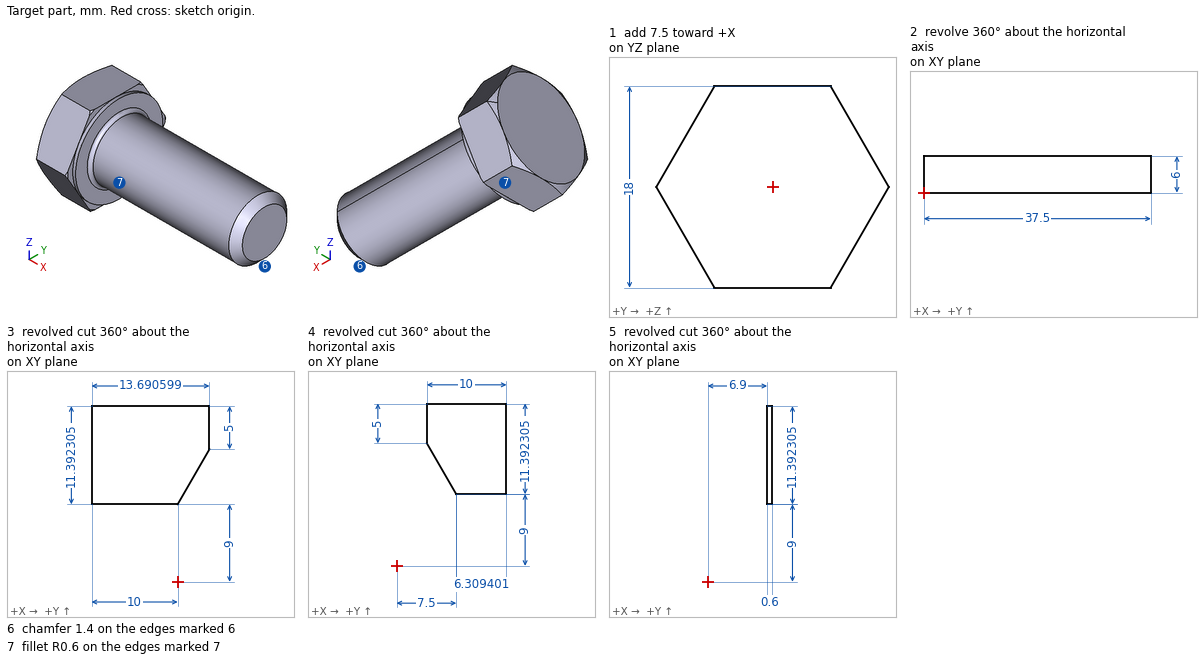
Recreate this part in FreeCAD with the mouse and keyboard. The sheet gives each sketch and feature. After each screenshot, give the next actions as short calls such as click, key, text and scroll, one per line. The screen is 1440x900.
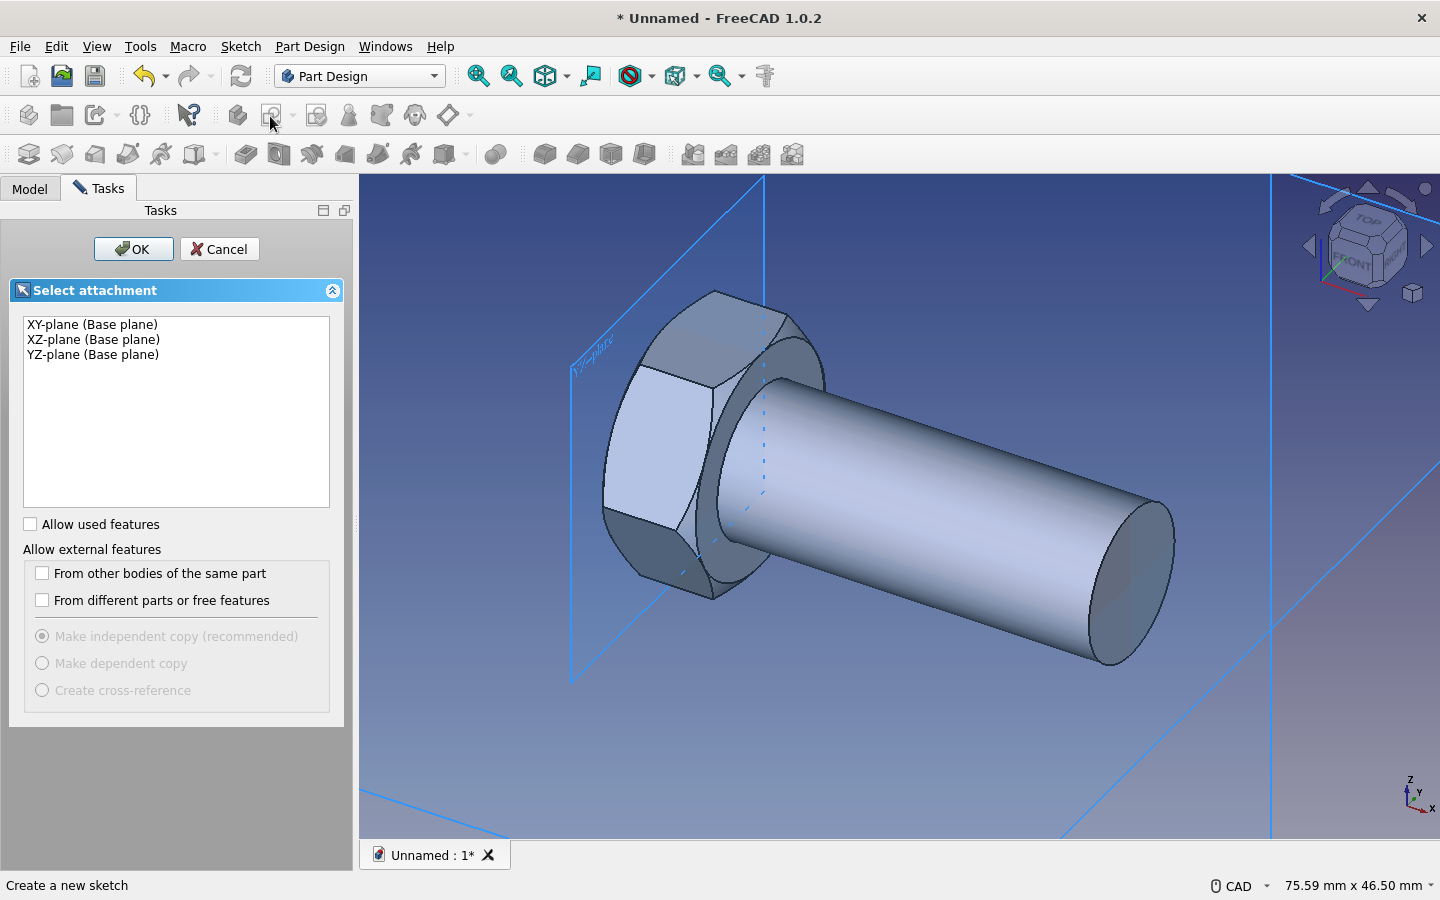
click(84, 324)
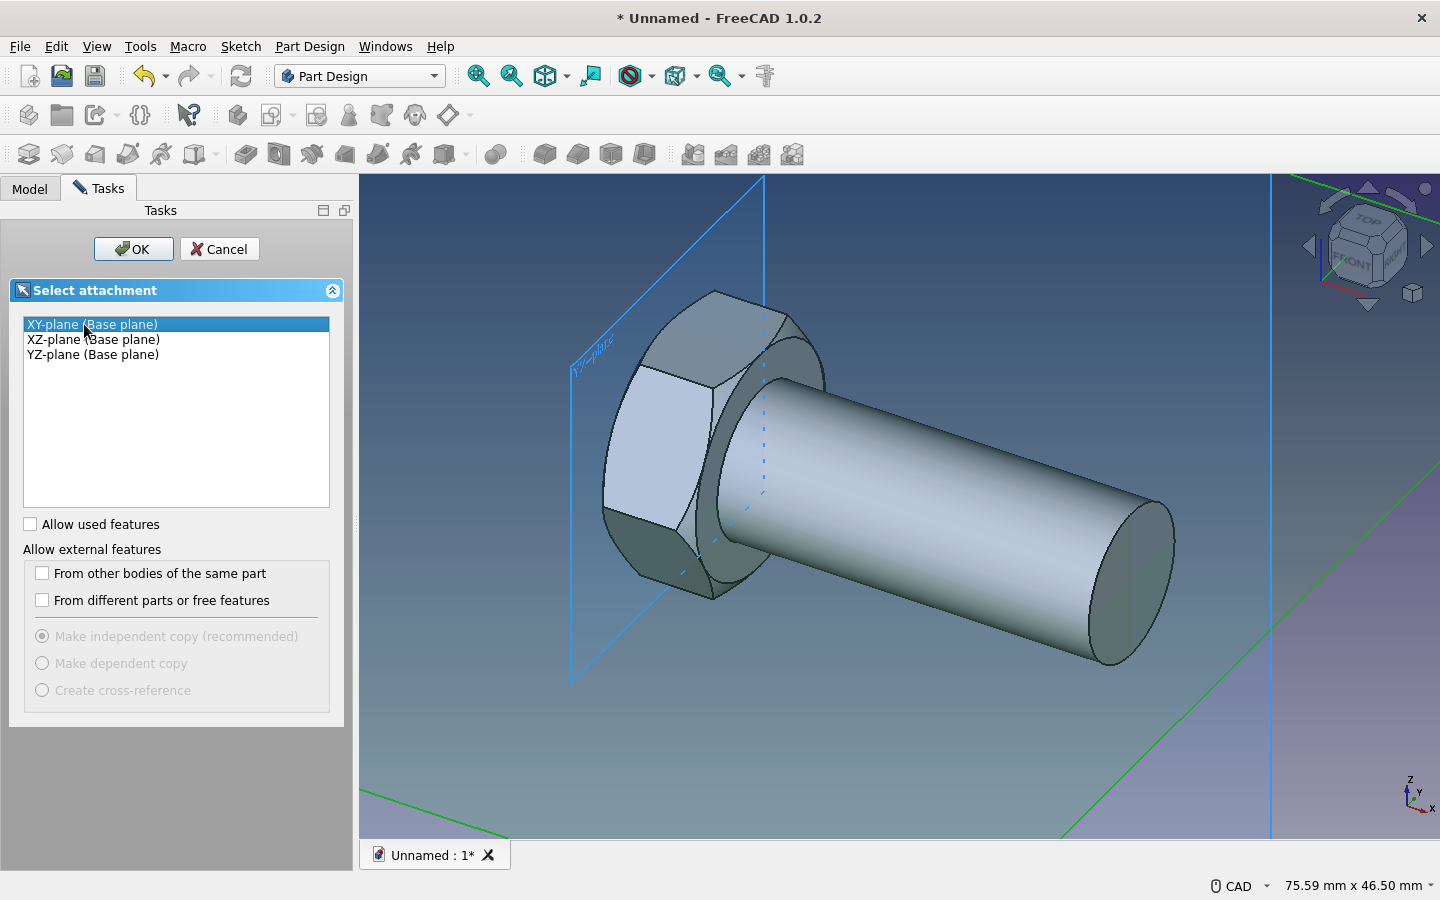
click(134, 249)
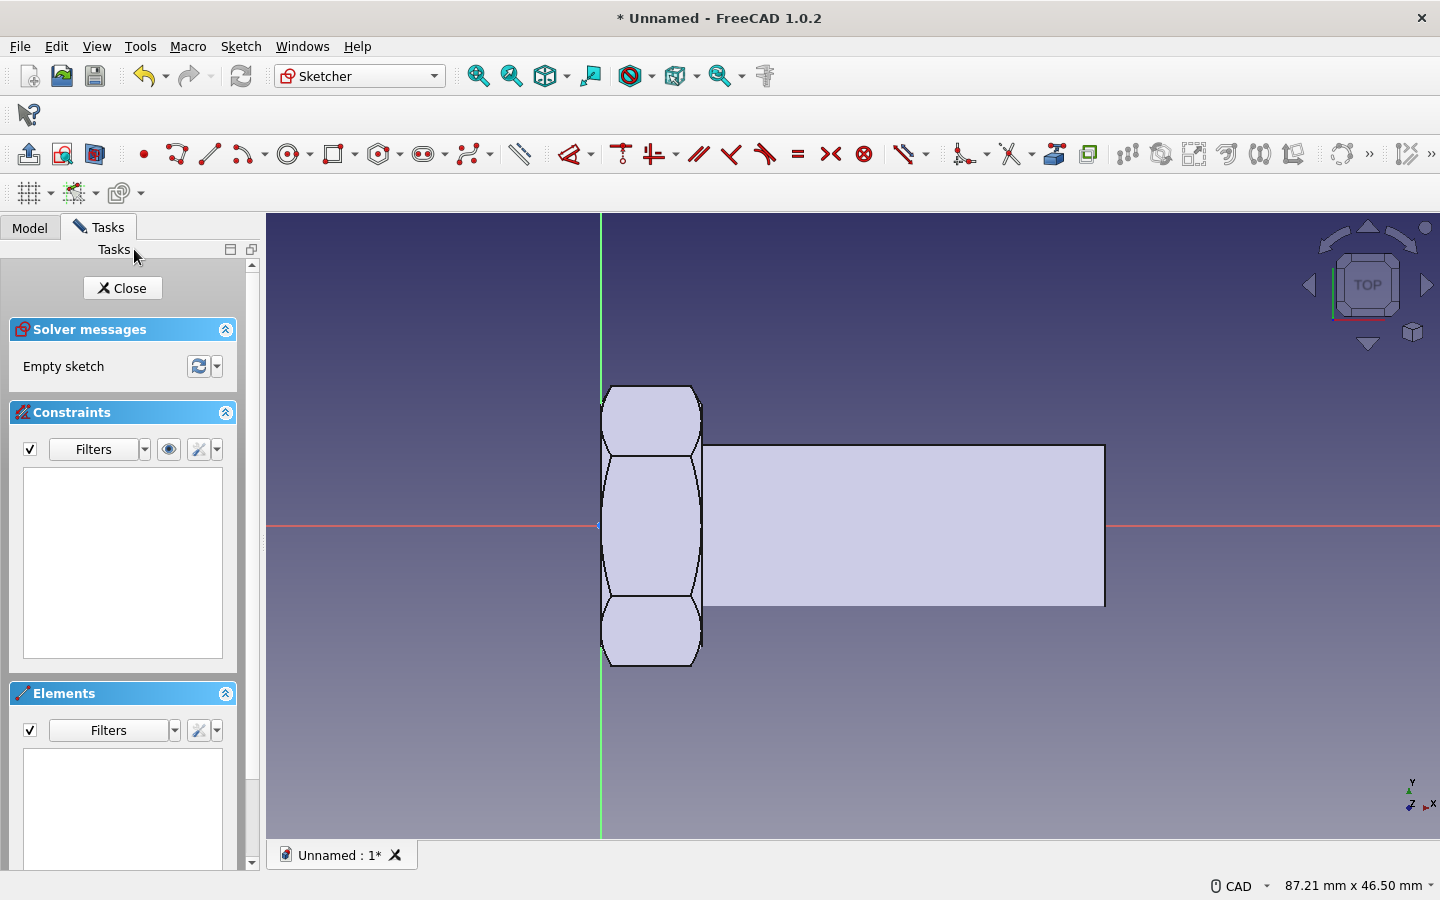
click(95, 154)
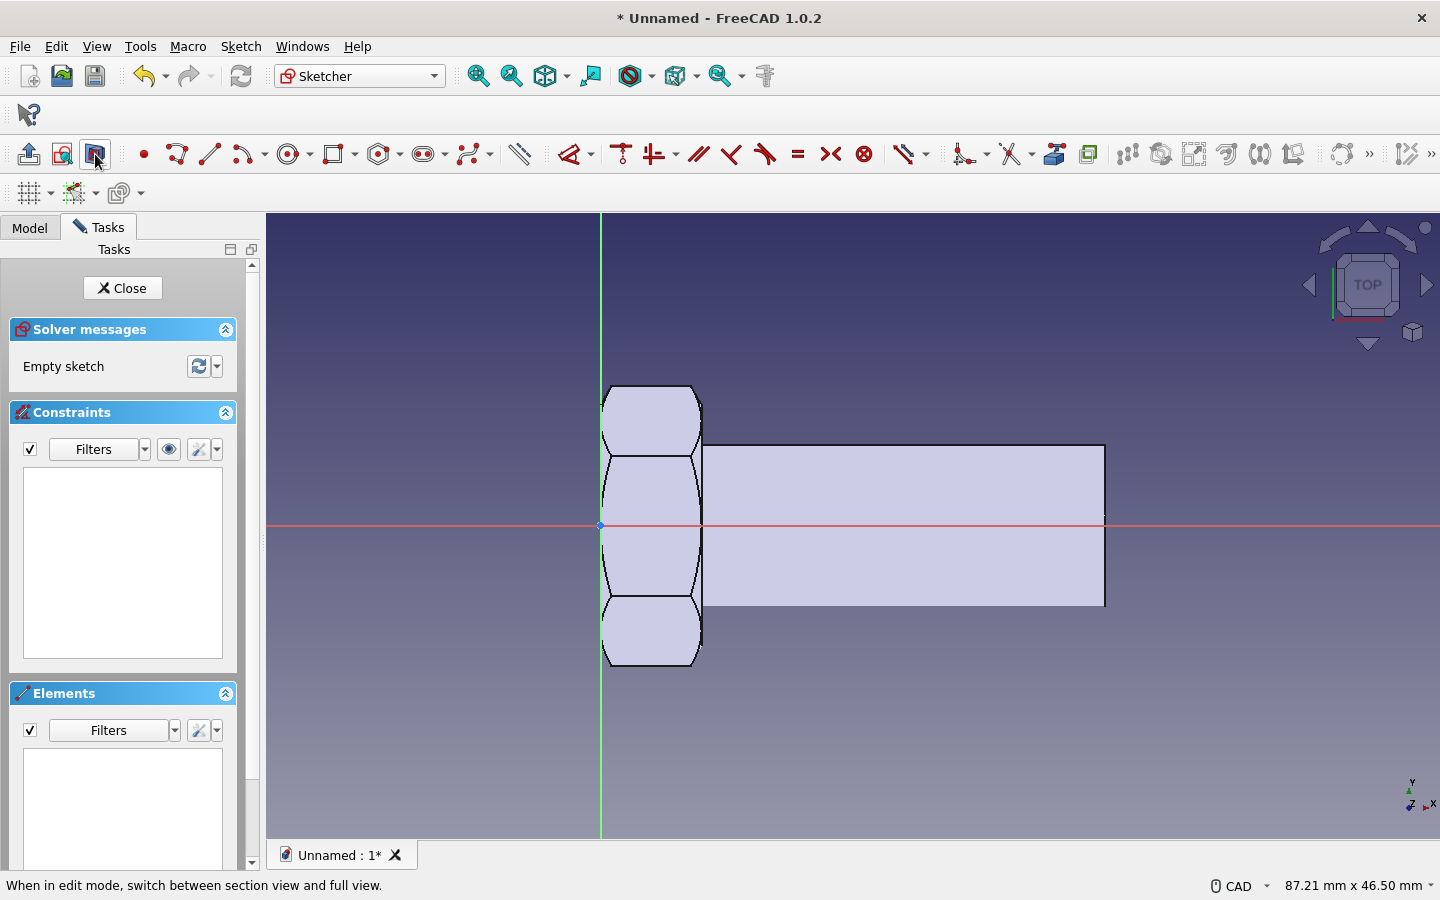
scroll(1275, 811, down, 1)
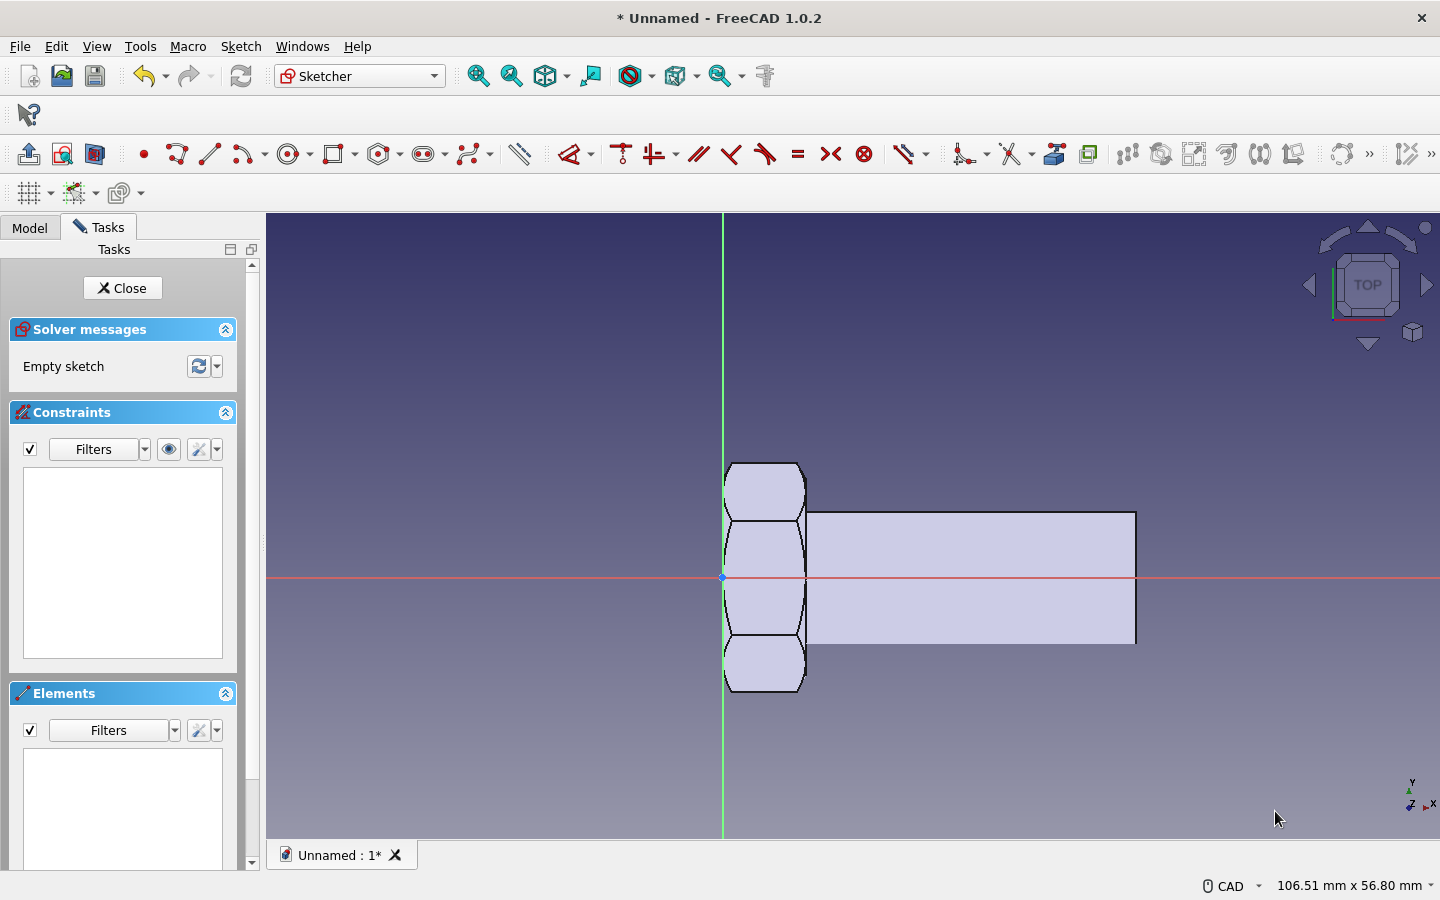
scroll(740, 392, up, 3)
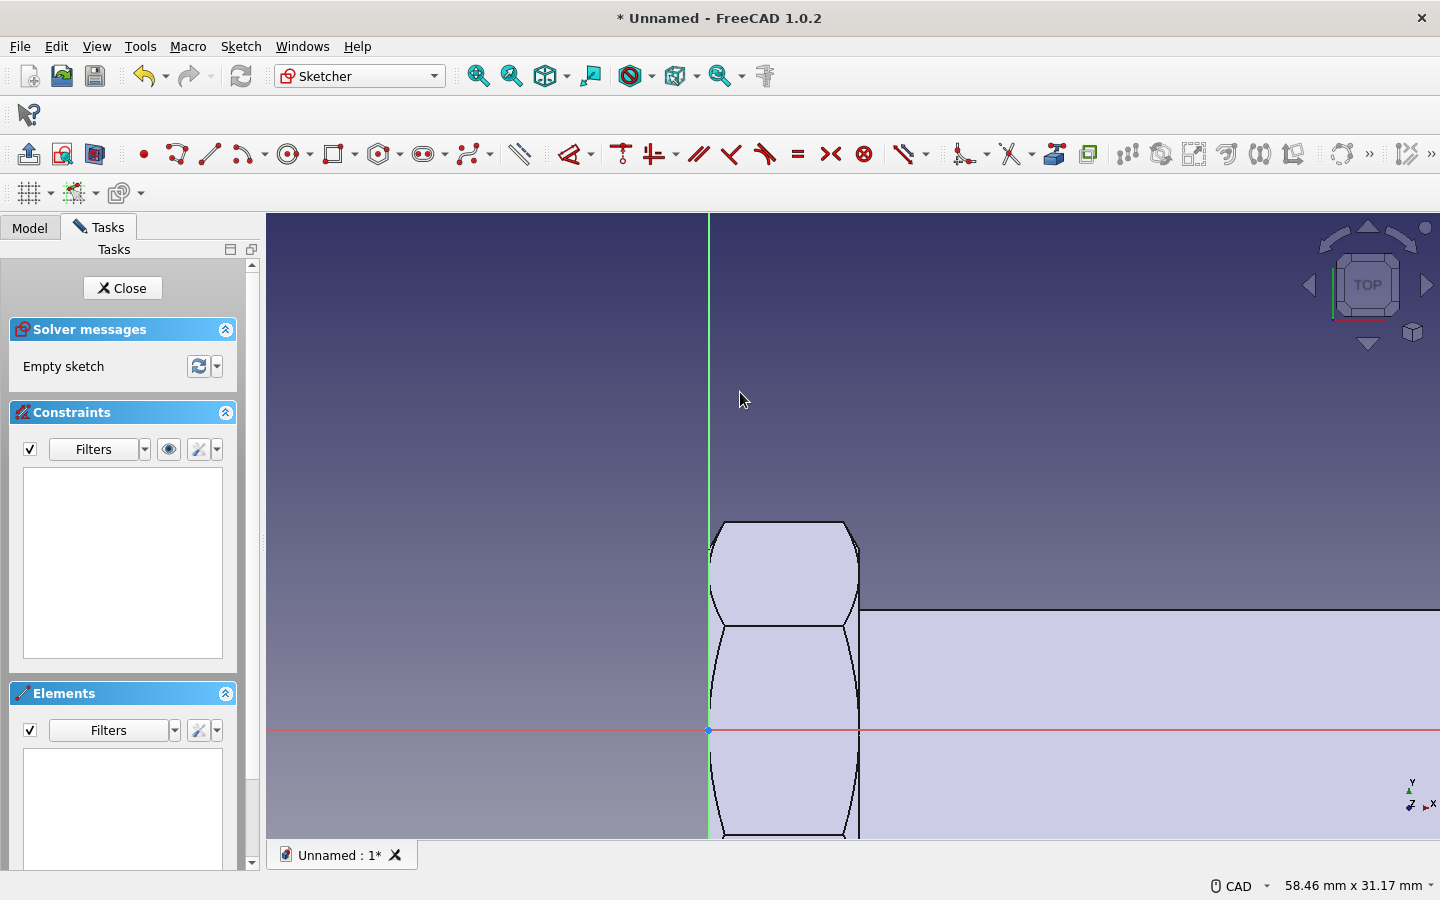
click(332, 154)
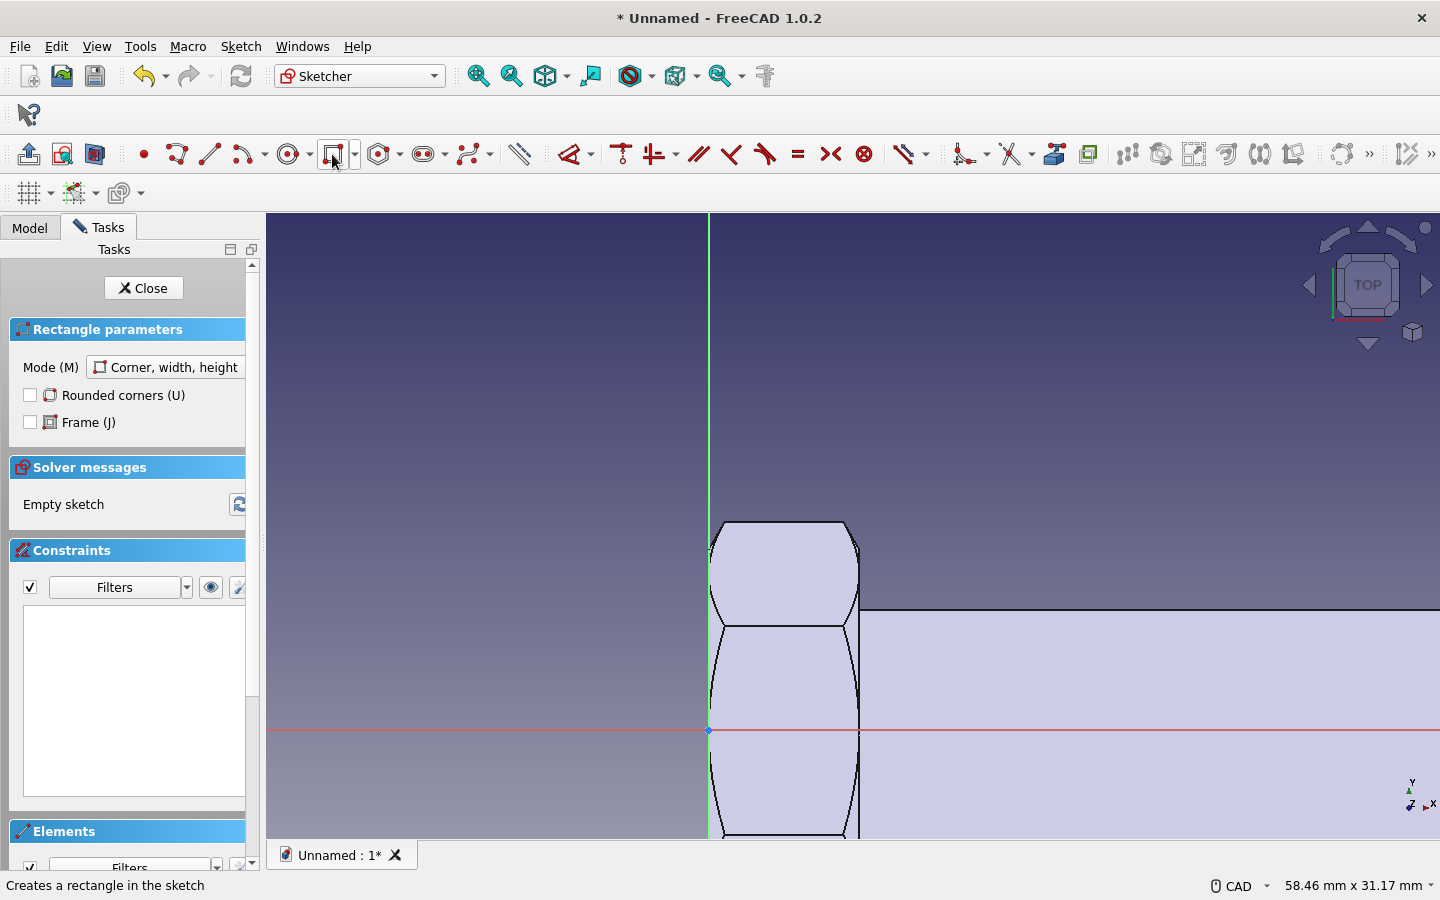
scroll(847, 321, up, 2)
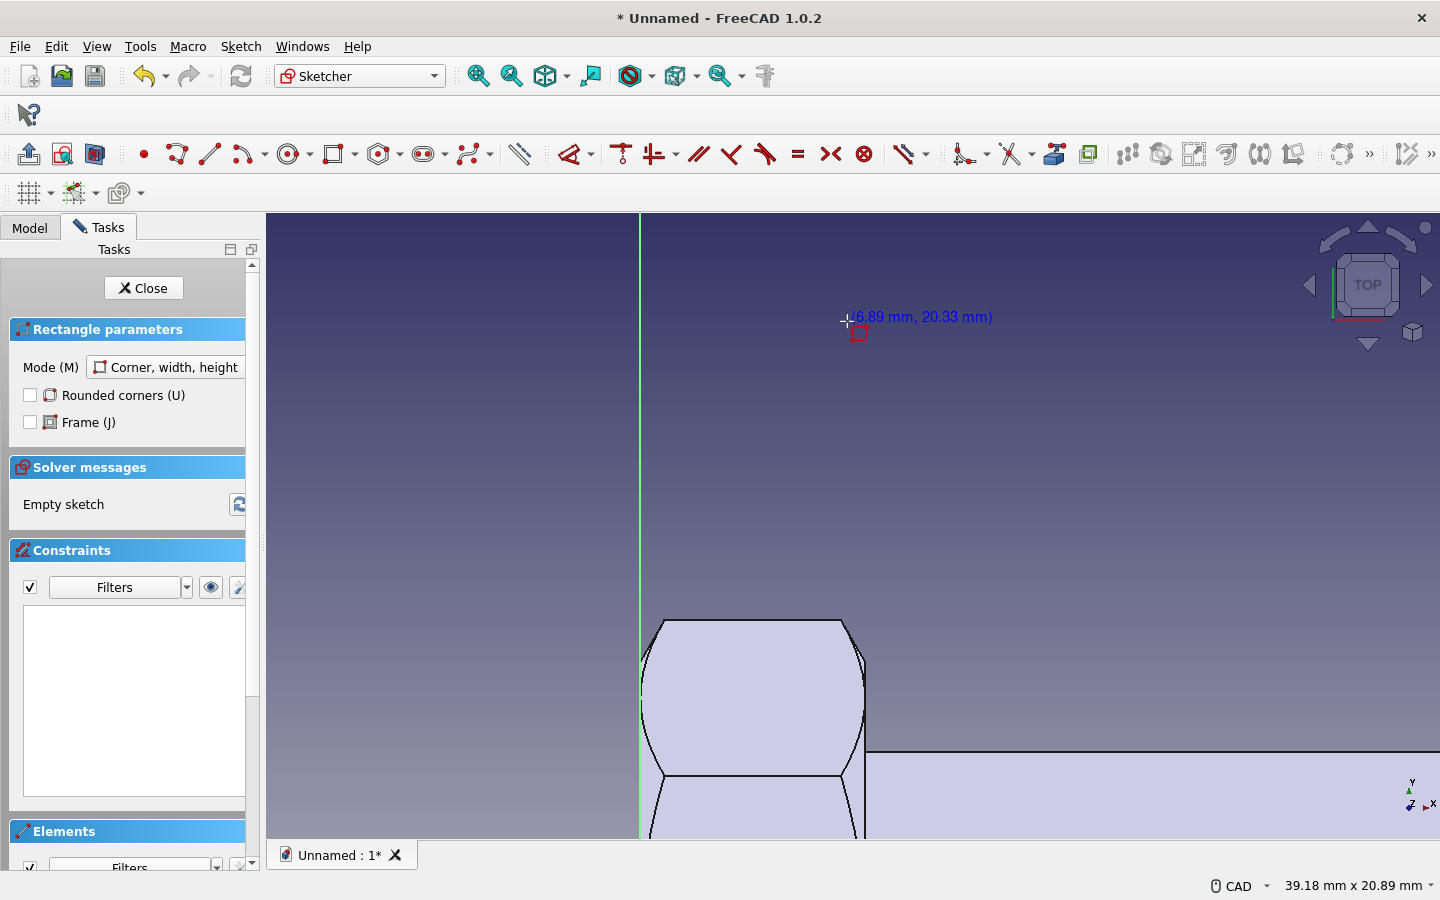
click(847, 321)
click(865, 662)
key(Escape)